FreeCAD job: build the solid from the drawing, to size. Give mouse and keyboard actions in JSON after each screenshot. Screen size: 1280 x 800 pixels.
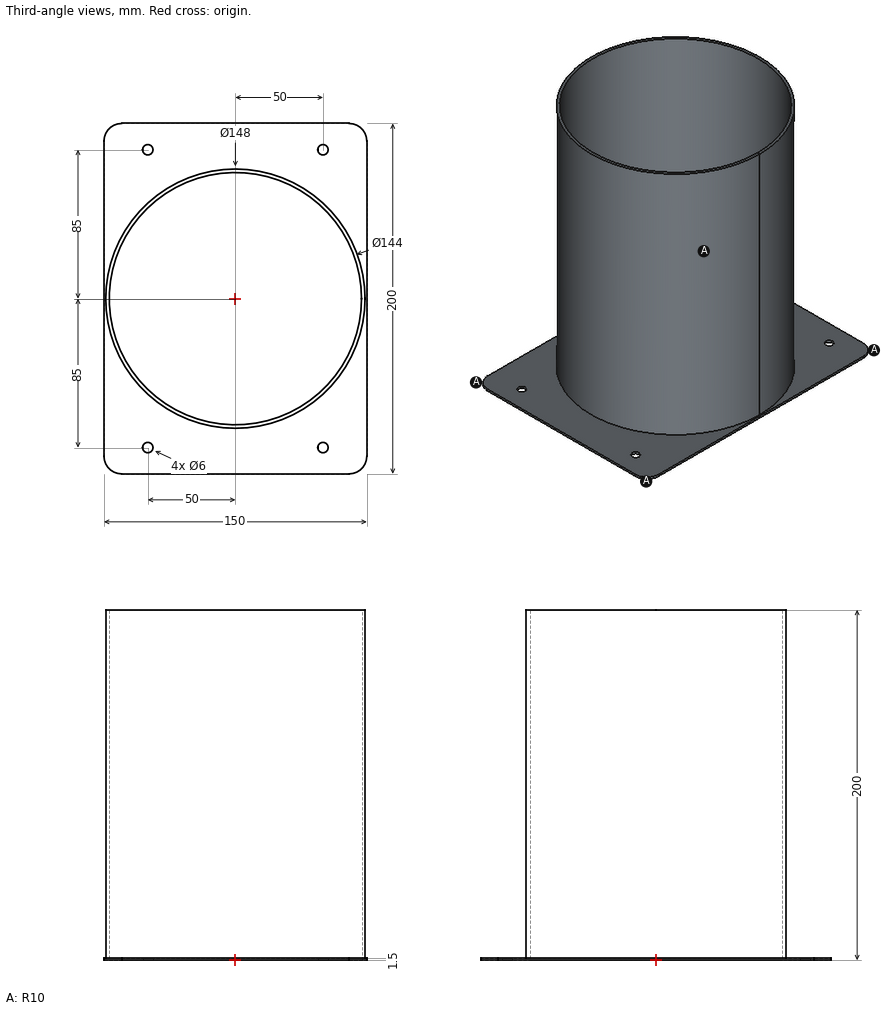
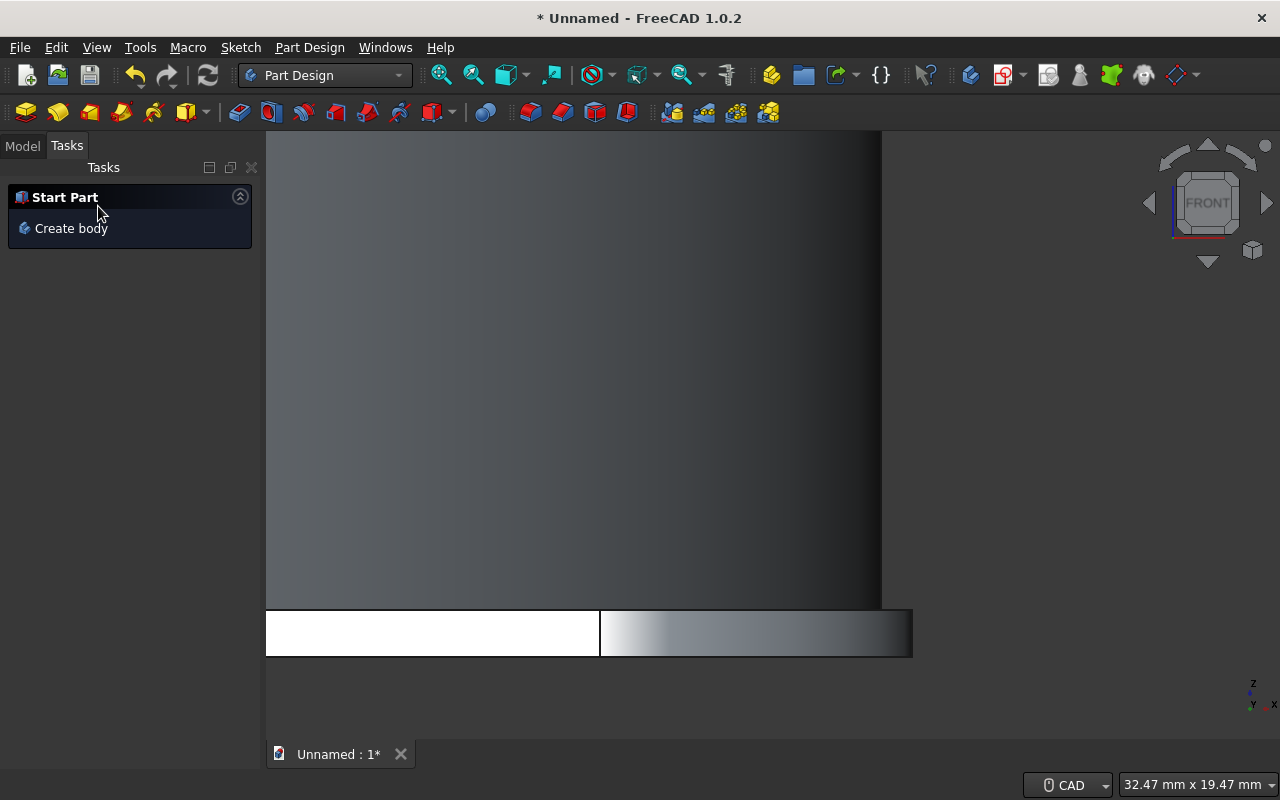
{"action": "left_click", "coordinate": [442, 76]}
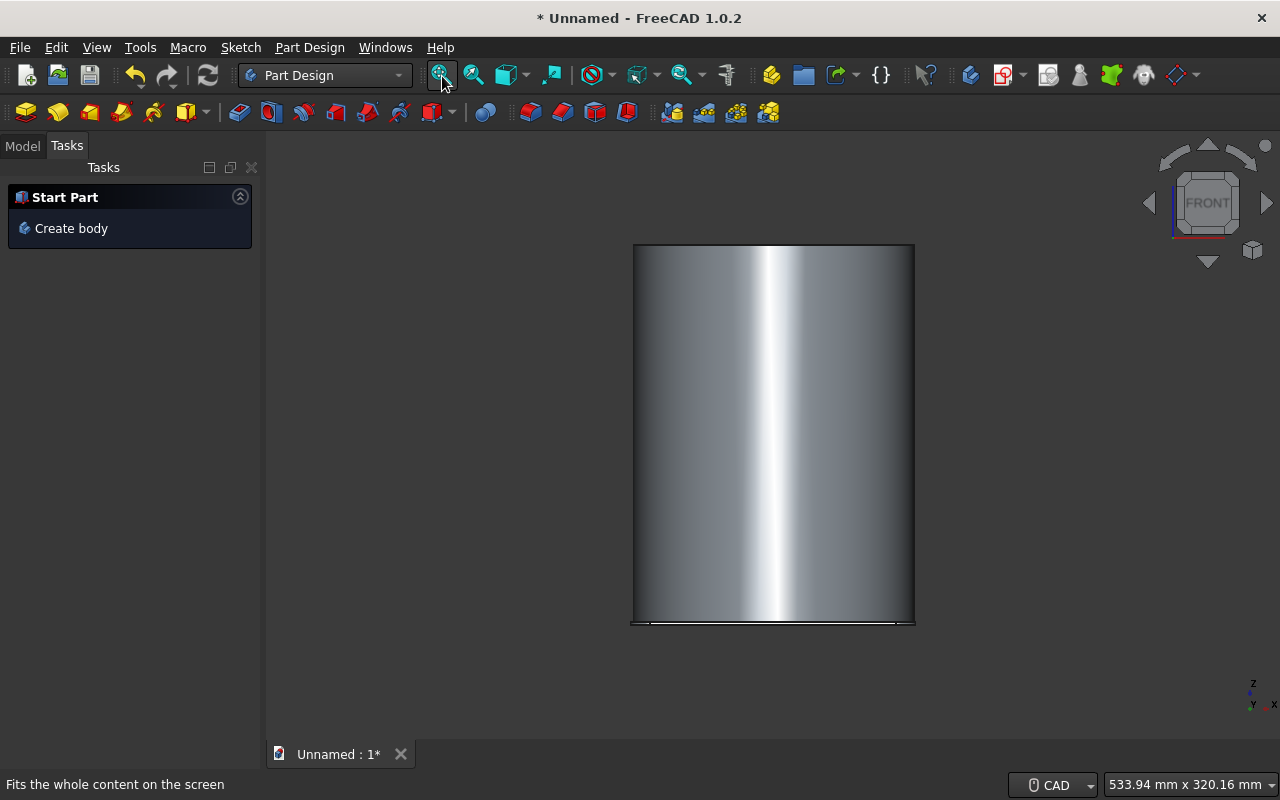
{"action": "key", "text": "0"}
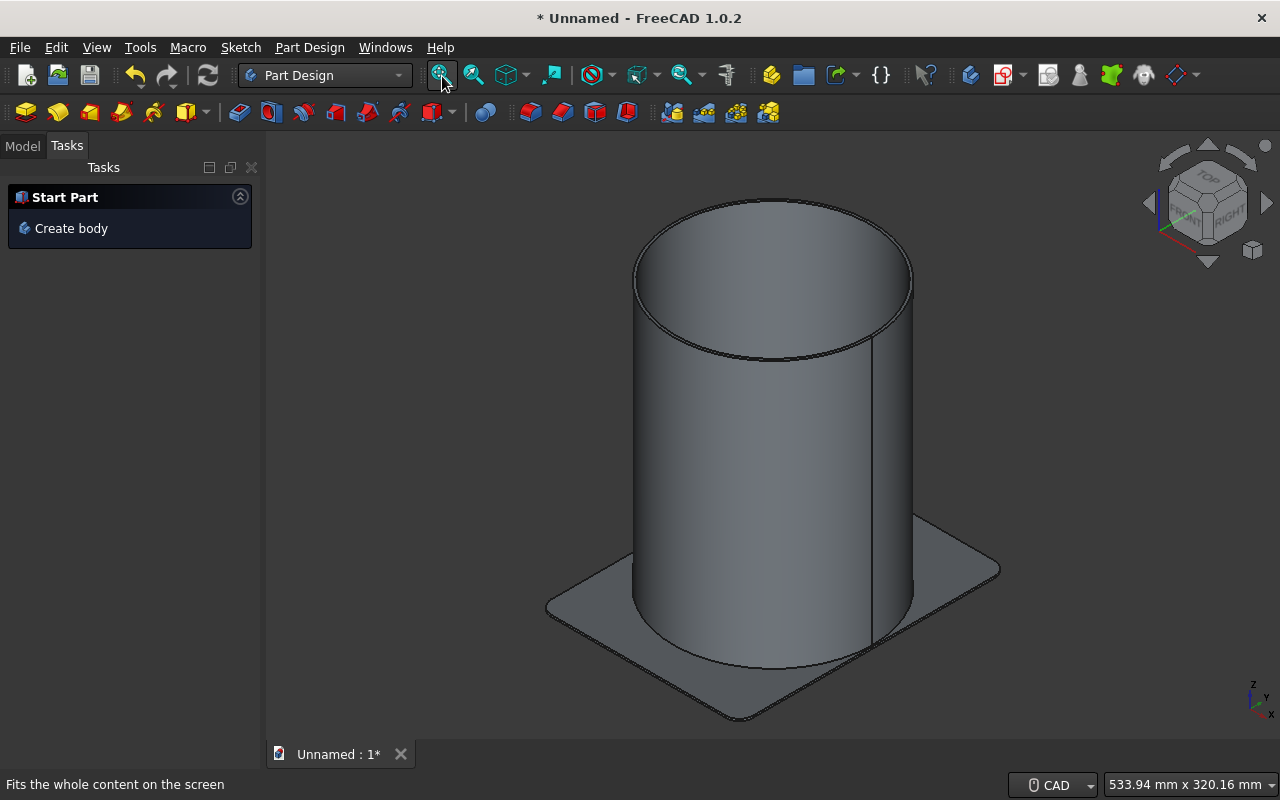
{"action": "left_click", "coordinate": [715, 686]}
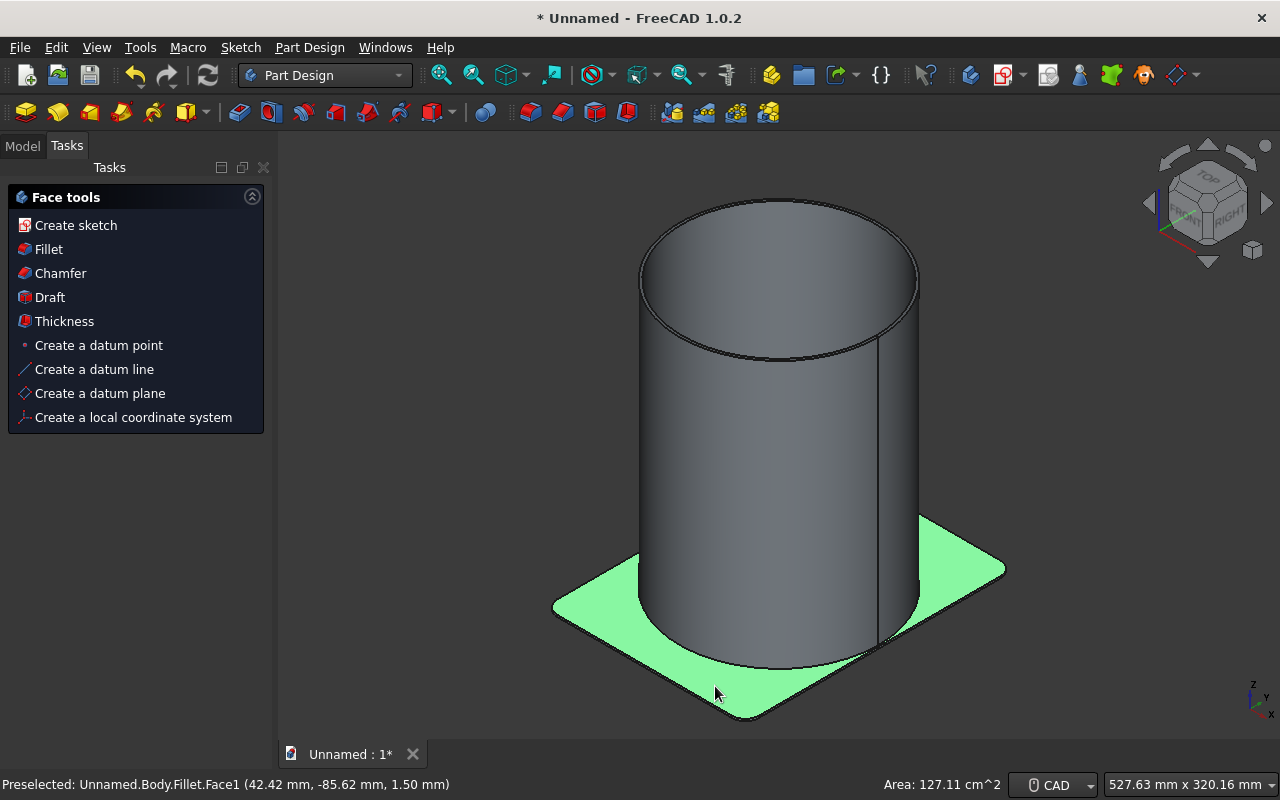
{"action": "left_click", "coordinate": [1004, 76]}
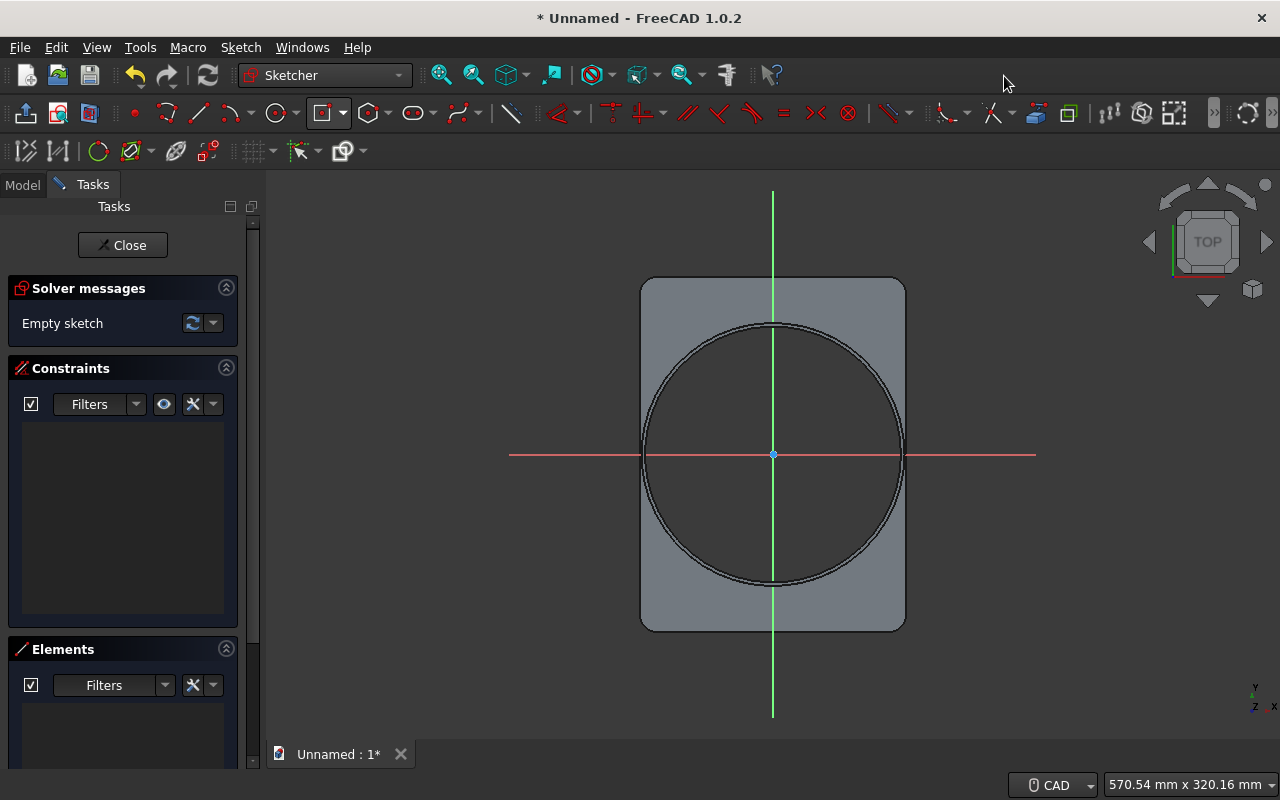
{"action": "left_click", "coordinate": [90, 114]}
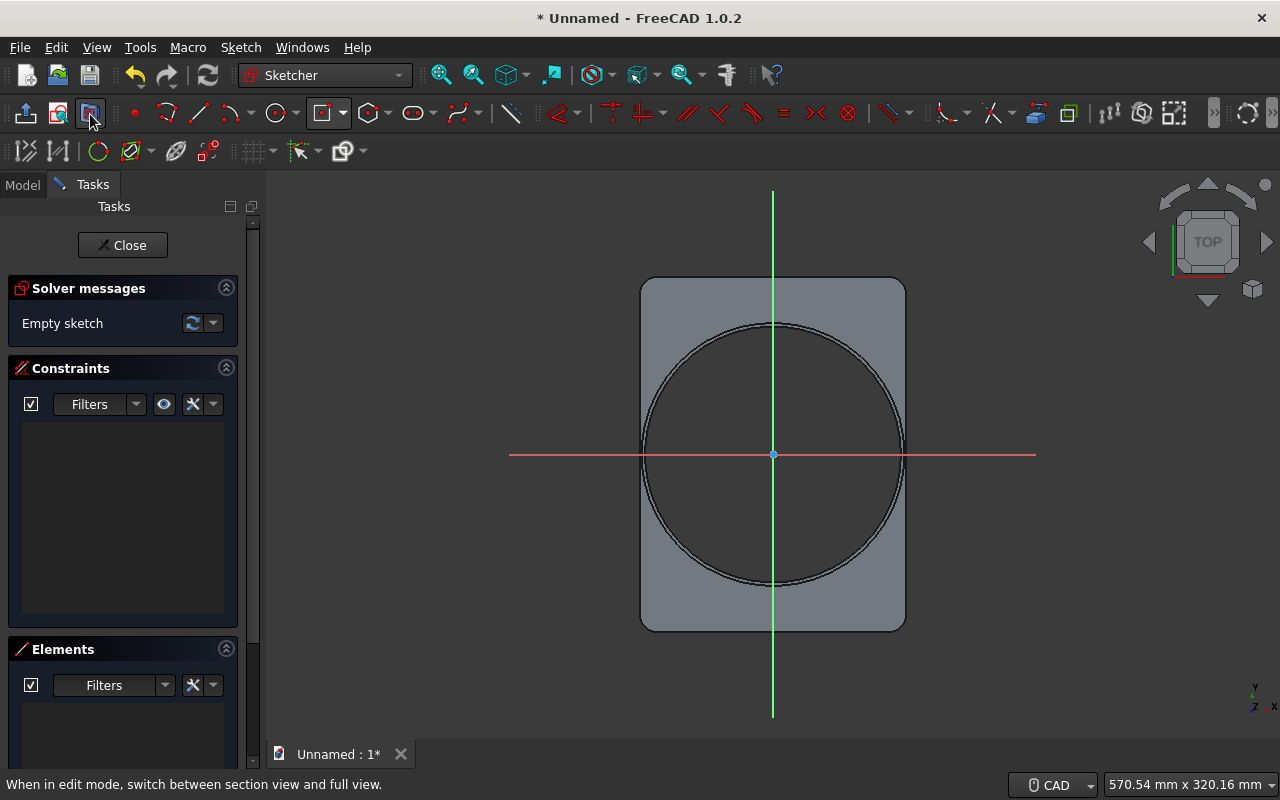
{"action": "left_click", "coordinate": [276, 114]}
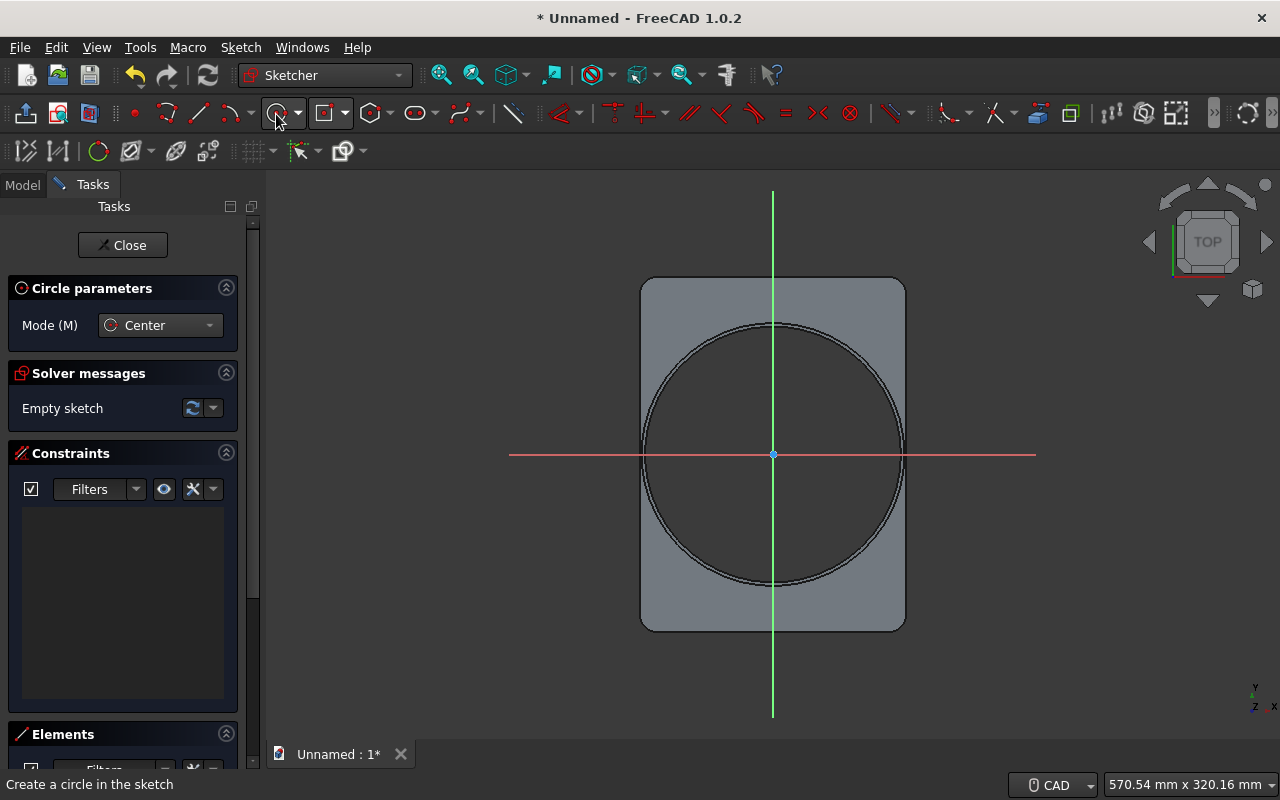
{"action": "scroll", "coordinate": [684, 606], "scroll_direction": "up", "scroll_amount": 8}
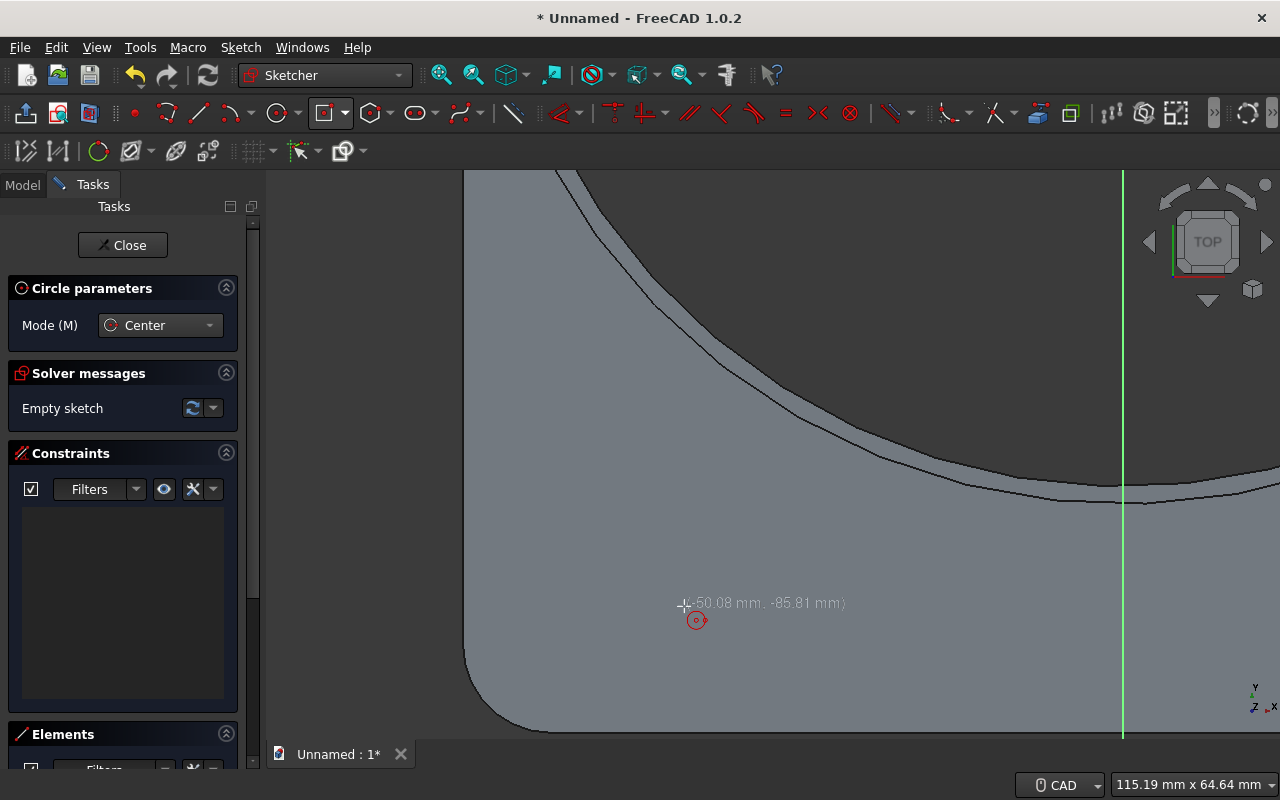
{"action": "scroll", "coordinate": [567, 652], "scroll_direction": "down", "scroll_amount": 7}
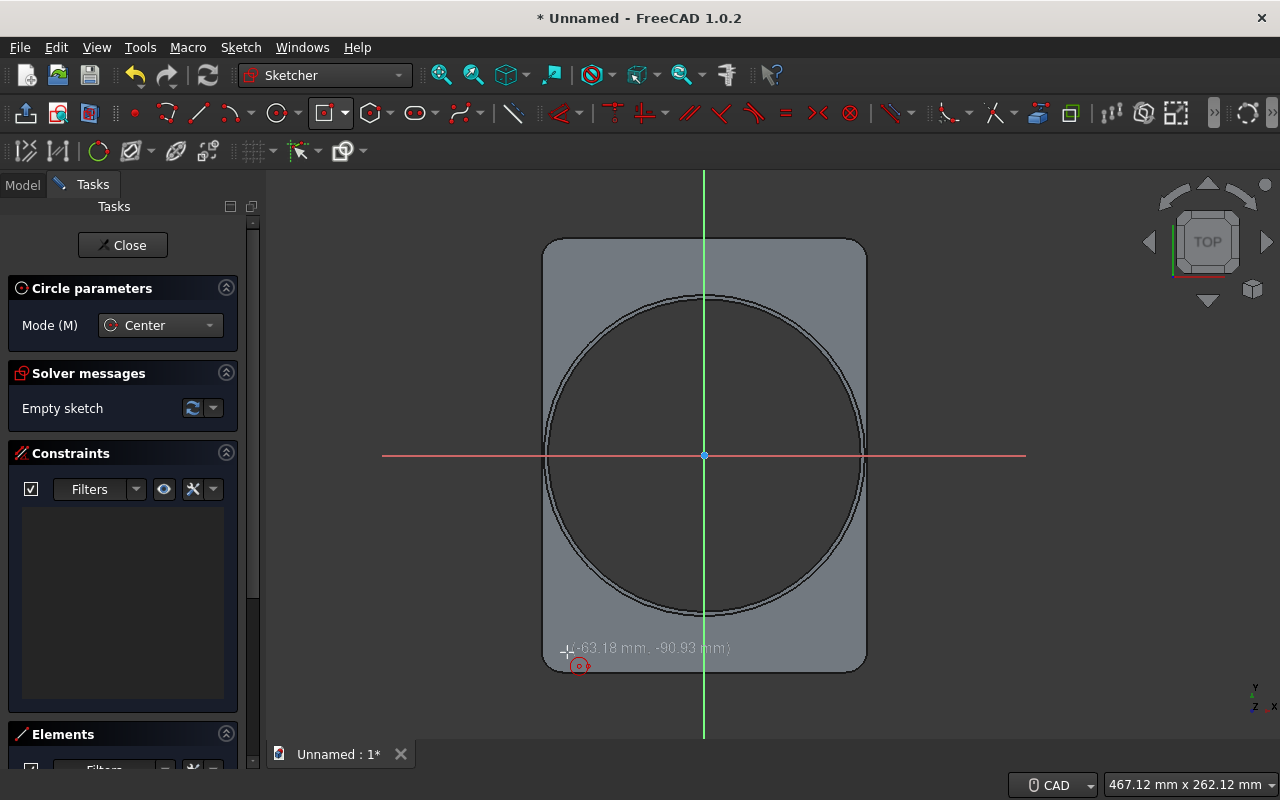
{"action": "left_click", "coordinate": [596, 640]}
{"action": "mouse_move", "coordinate": [600, 635]}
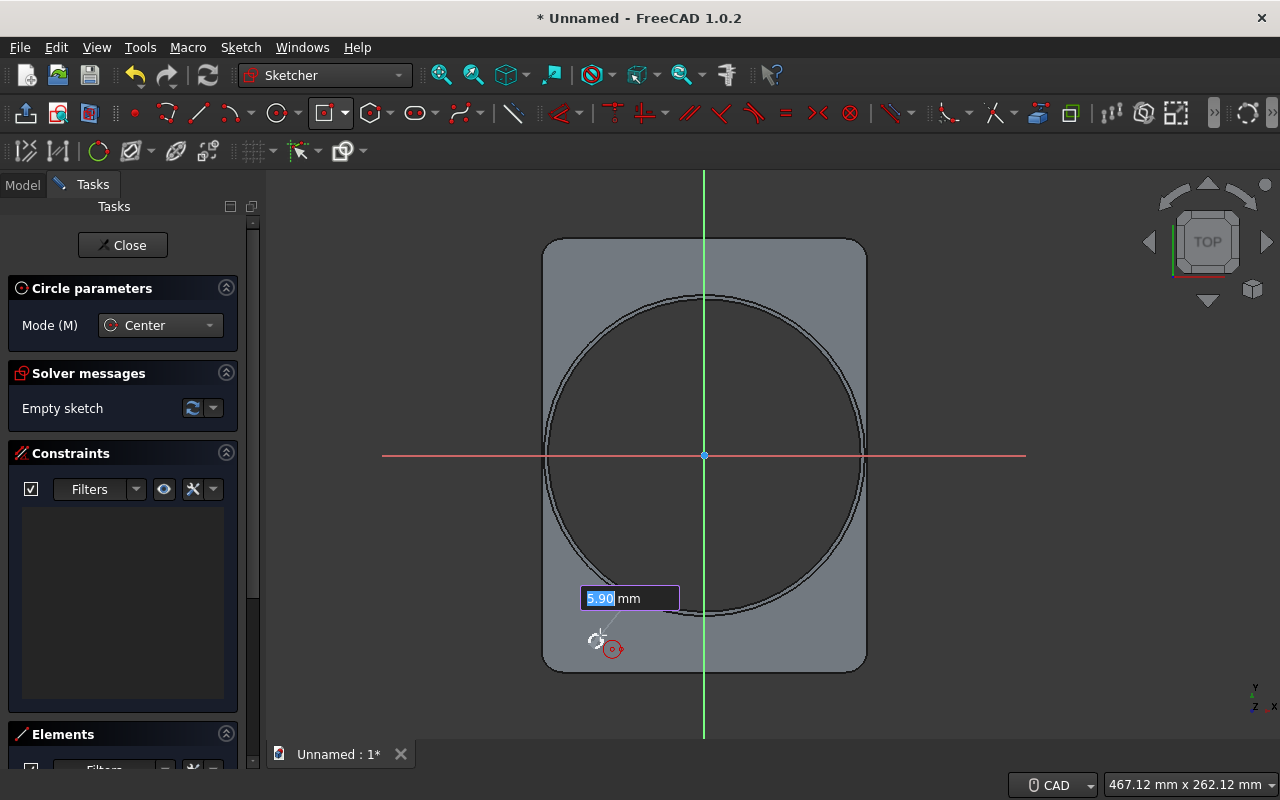
{"action": "type", "text": "6"}
{"action": "key", "text": "Return"}